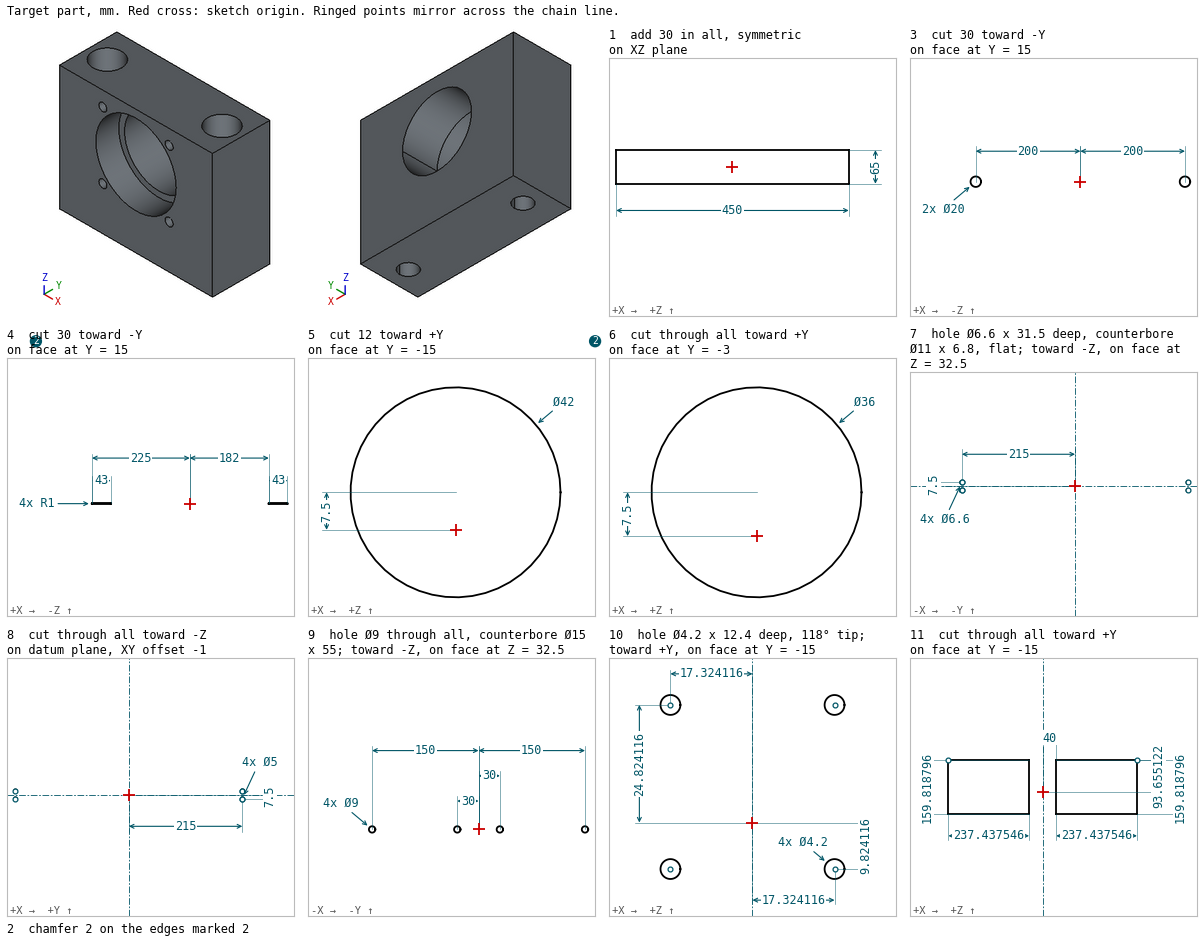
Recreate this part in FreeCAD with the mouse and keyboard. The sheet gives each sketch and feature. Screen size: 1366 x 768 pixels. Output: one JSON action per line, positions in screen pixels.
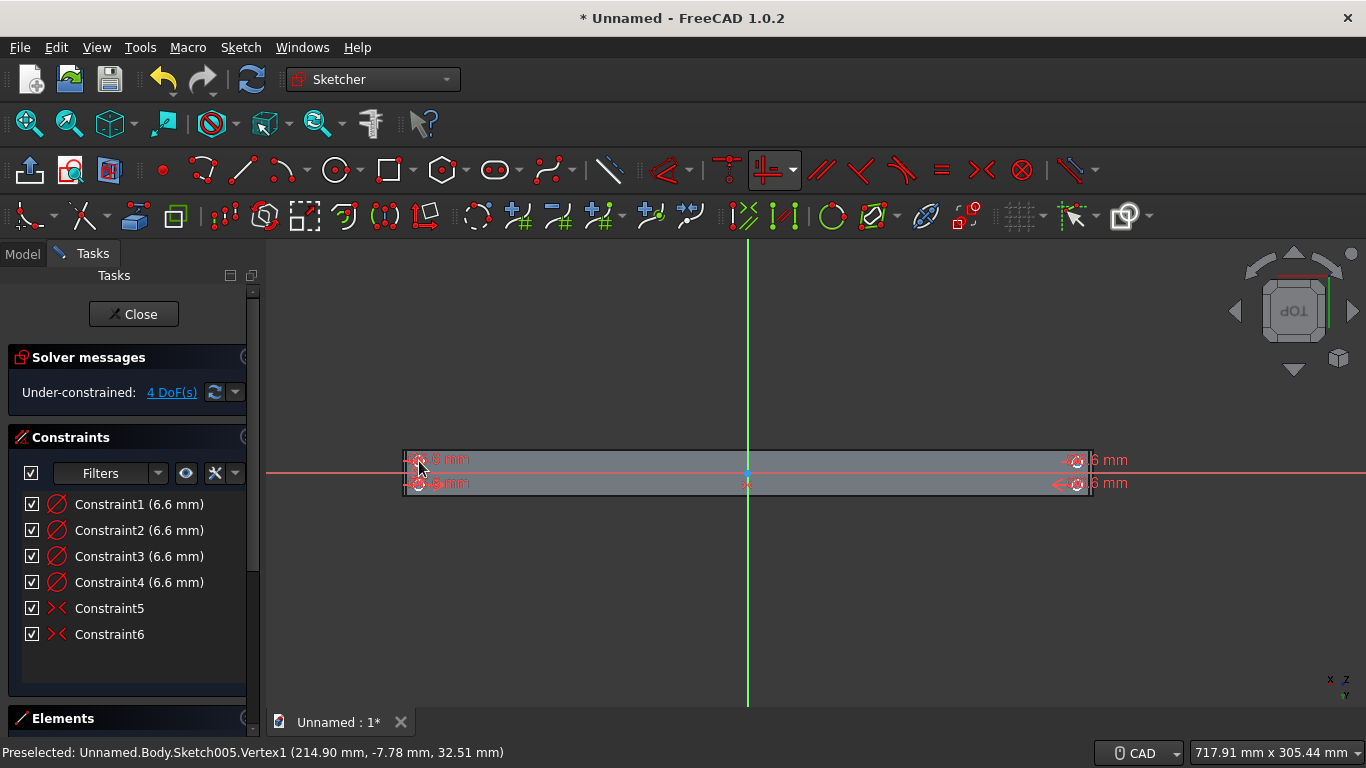
{"action": "left_click", "coordinate": [1077, 462]}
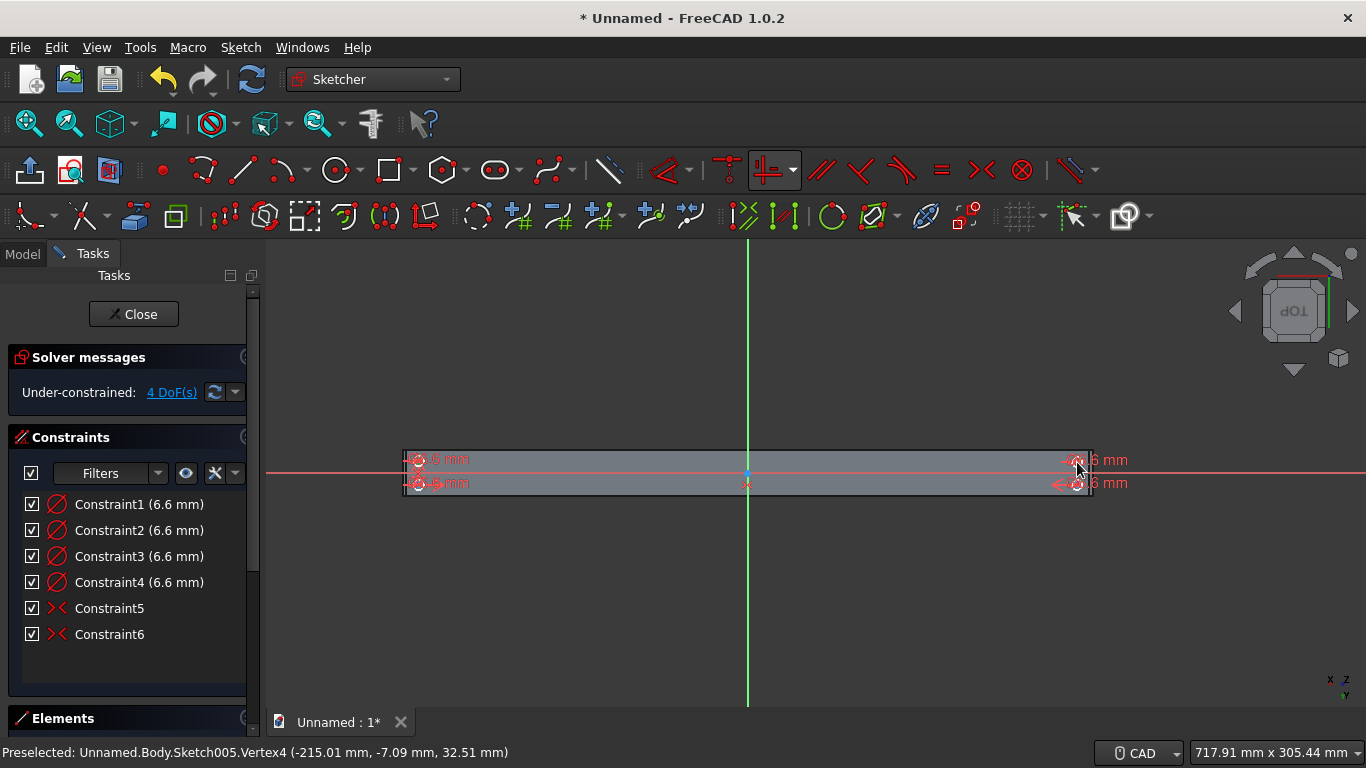
{"action": "left_click", "coordinate": [748, 650]}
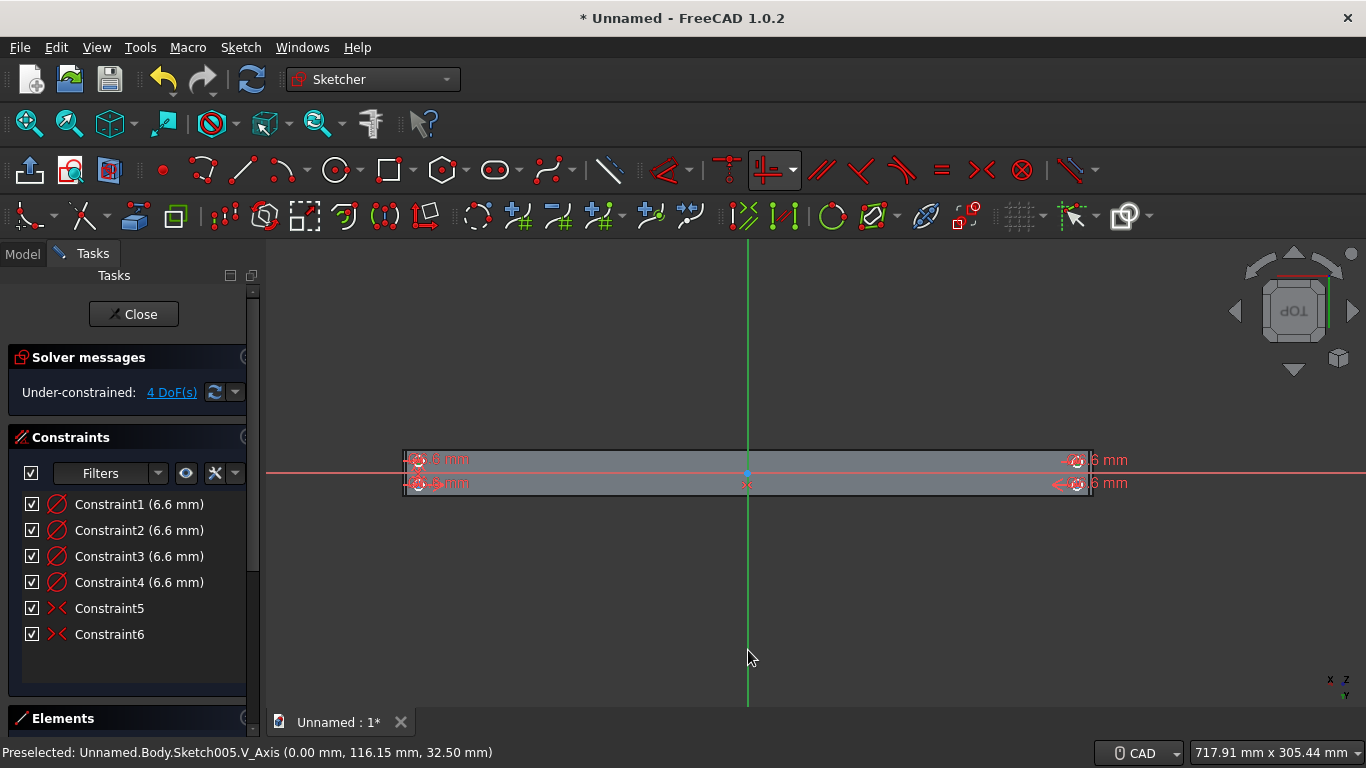
{"action": "key", "text": "s"}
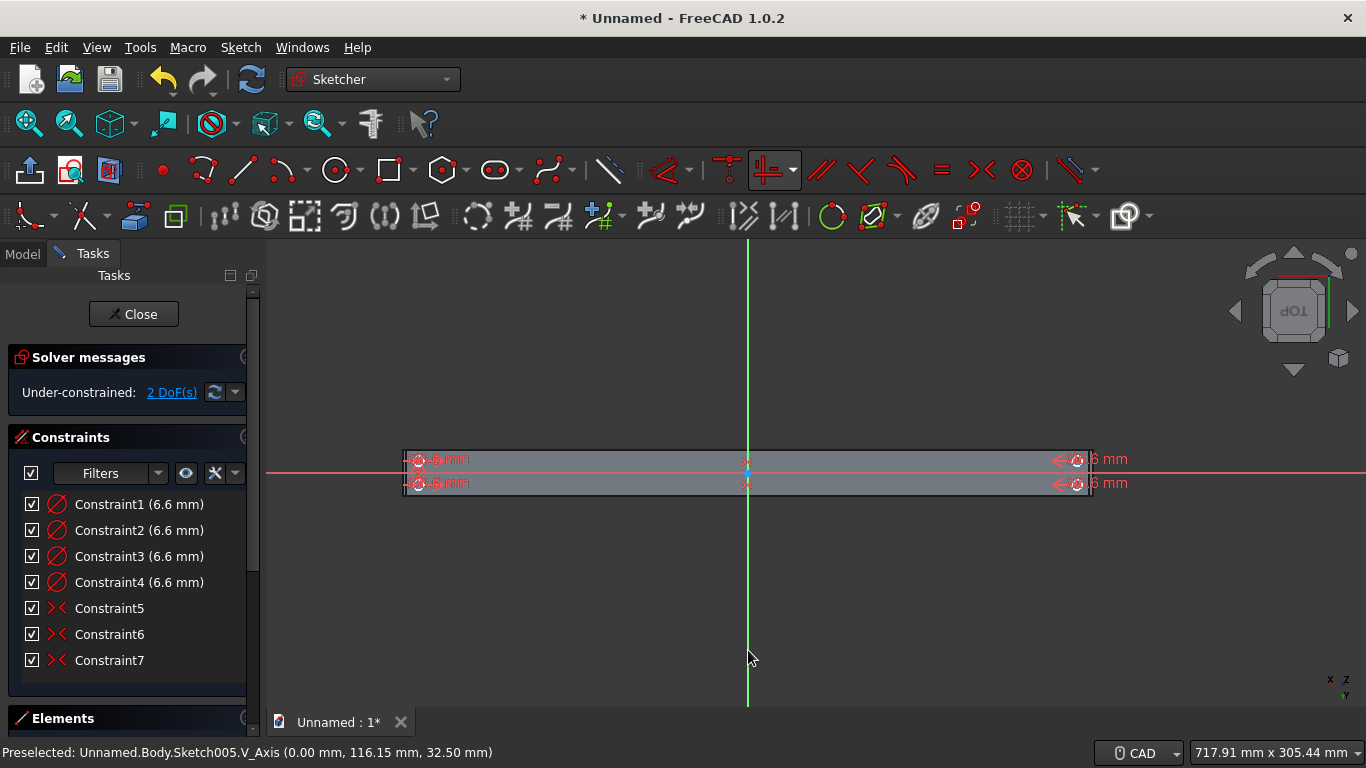
{"action": "key", "text": "d"}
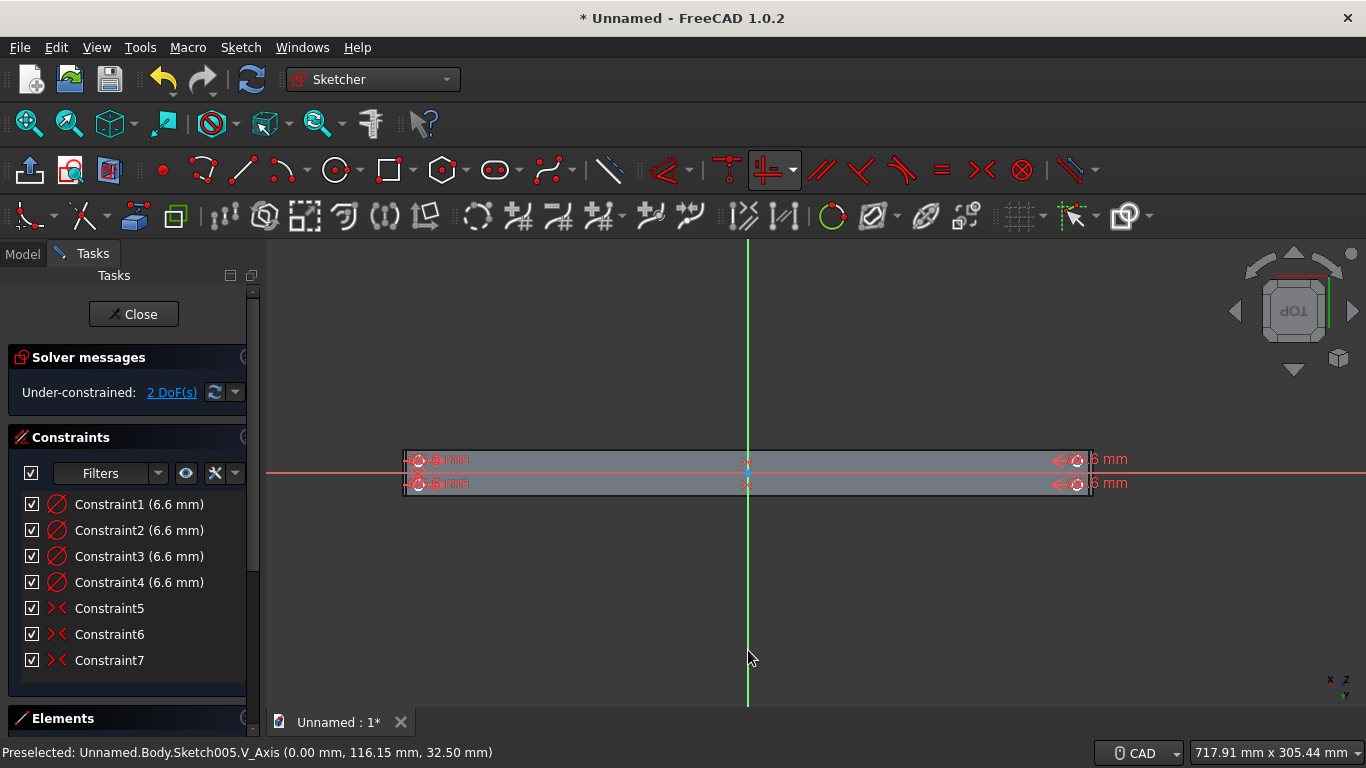
{"action": "left_click", "coordinate": [419, 461]}
{"action": "left_click", "coordinate": [583, 427]}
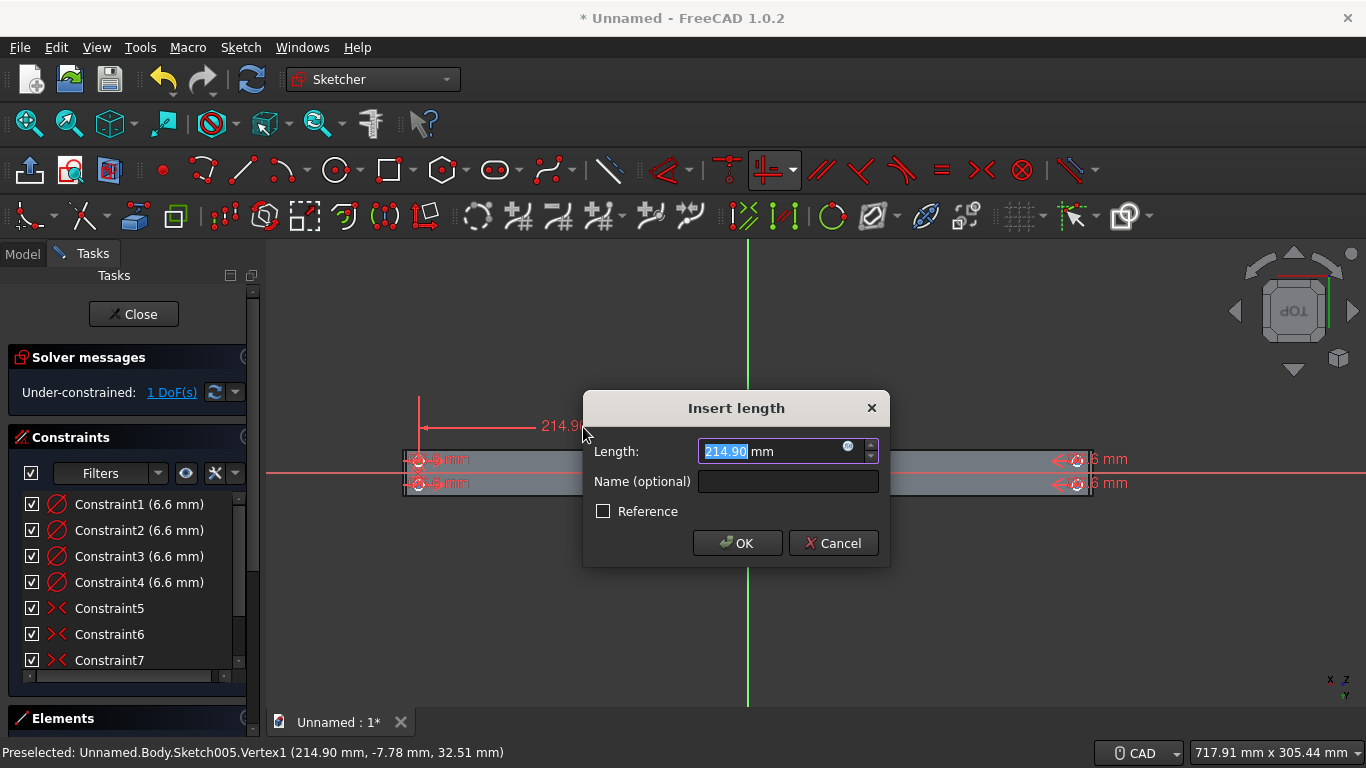
{"action": "type", "text": "215"}
{"action": "key", "text": "Return"}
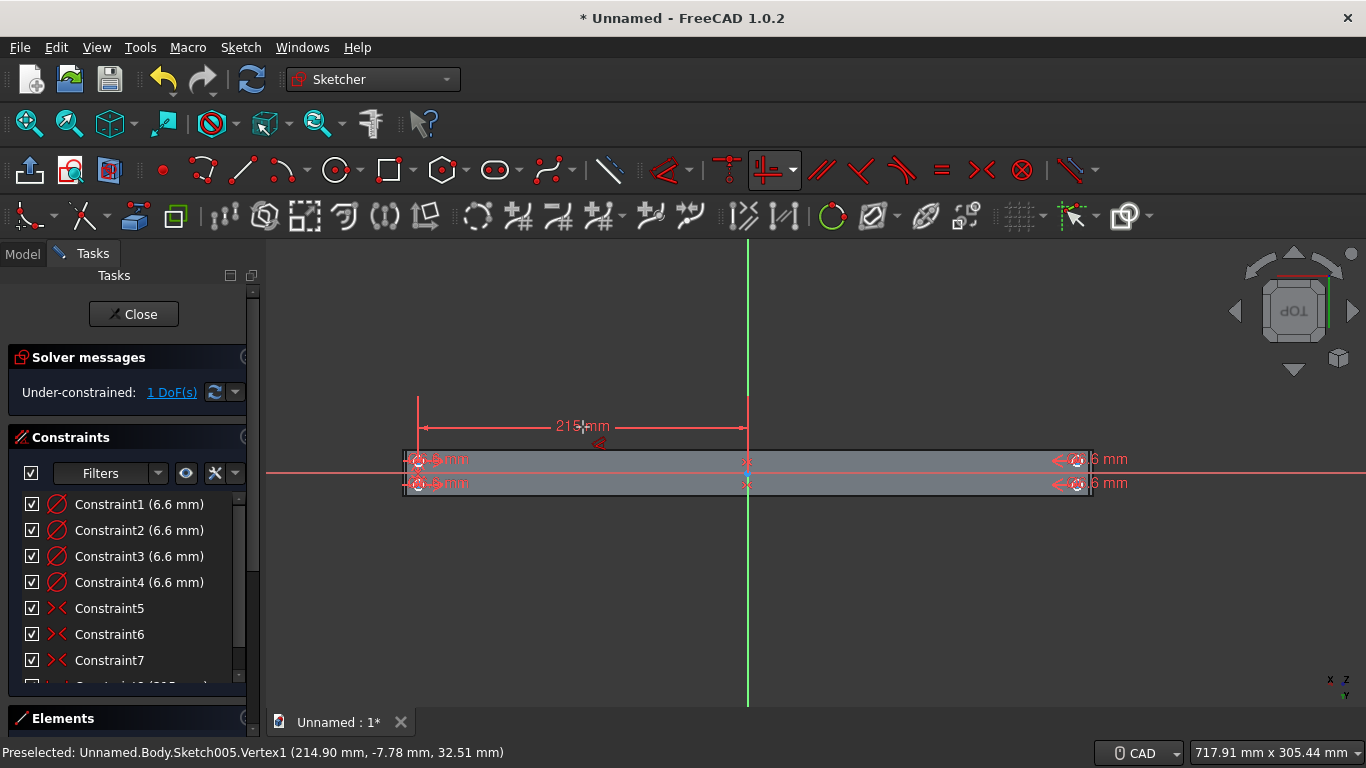
{"action": "scroll", "coordinate": [418, 461], "scroll_direction": "up", "scroll_amount": 7}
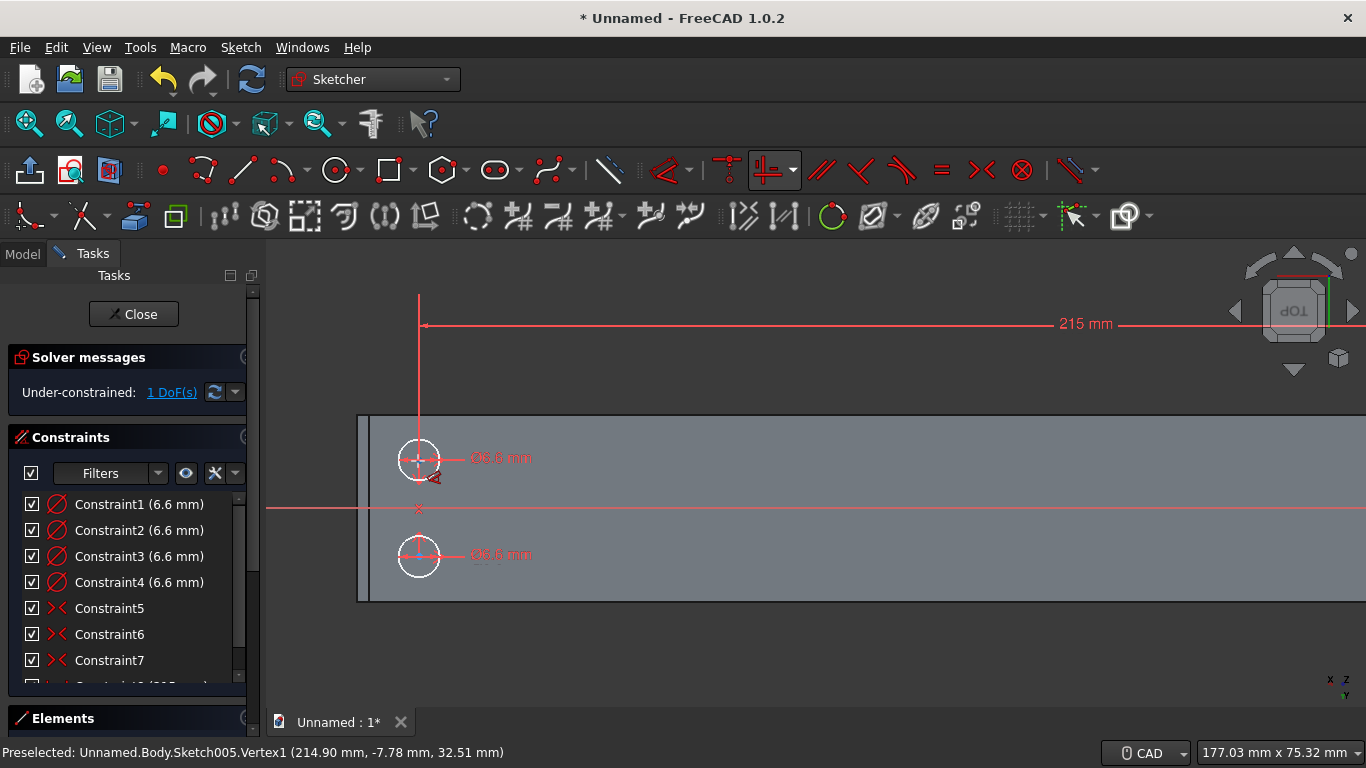
{"action": "left_click", "coordinate": [419, 460]}
{"action": "left_click", "coordinate": [385, 484]}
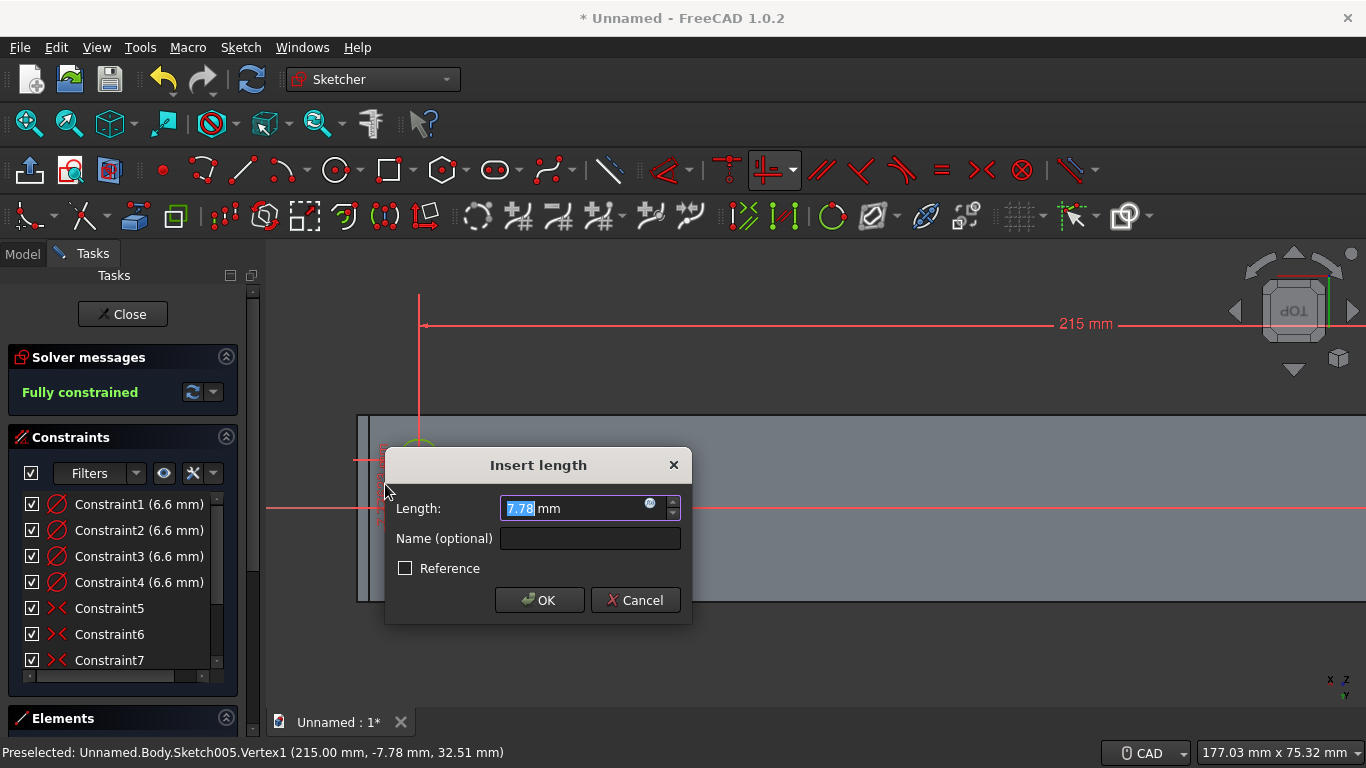
{"action": "type", "text": "7.5"}
{"action": "key", "text": "Return"}
{"action": "key", "text": "Escape"}